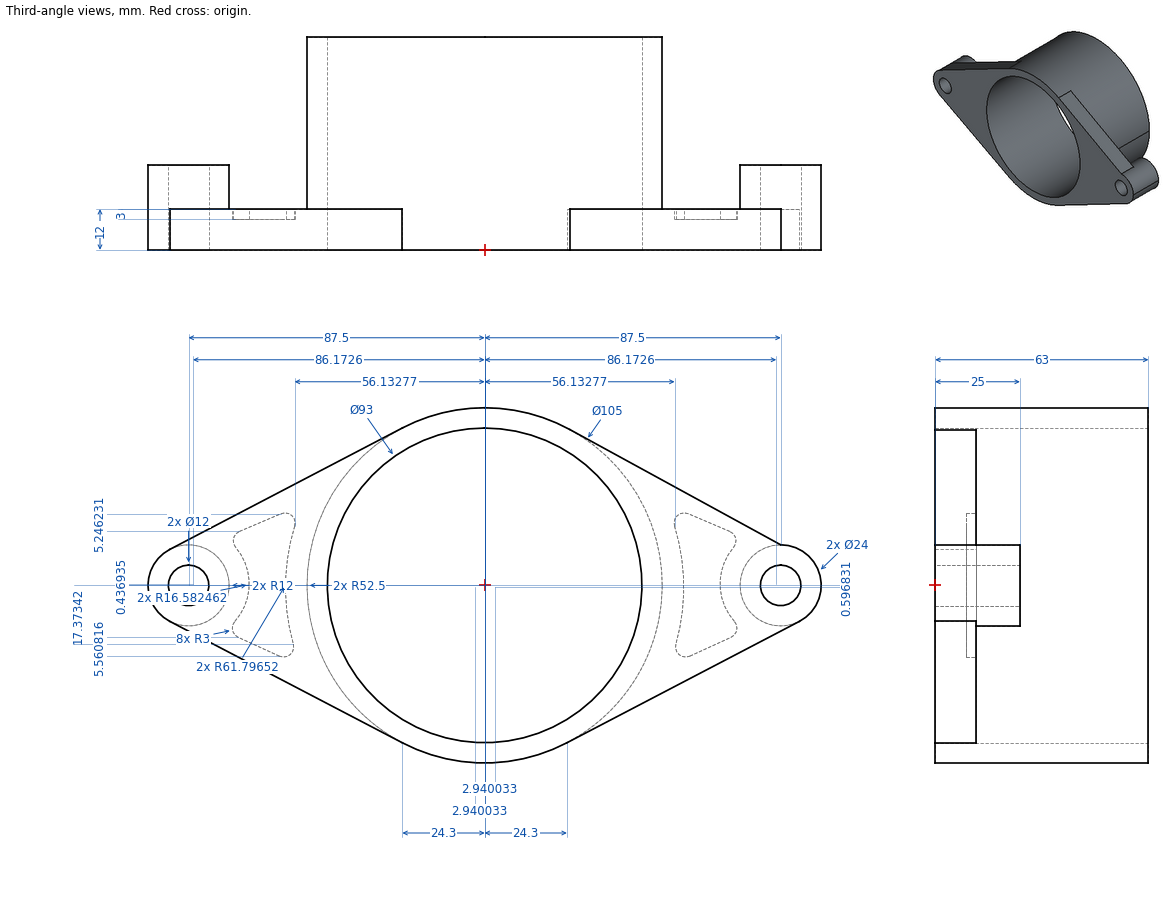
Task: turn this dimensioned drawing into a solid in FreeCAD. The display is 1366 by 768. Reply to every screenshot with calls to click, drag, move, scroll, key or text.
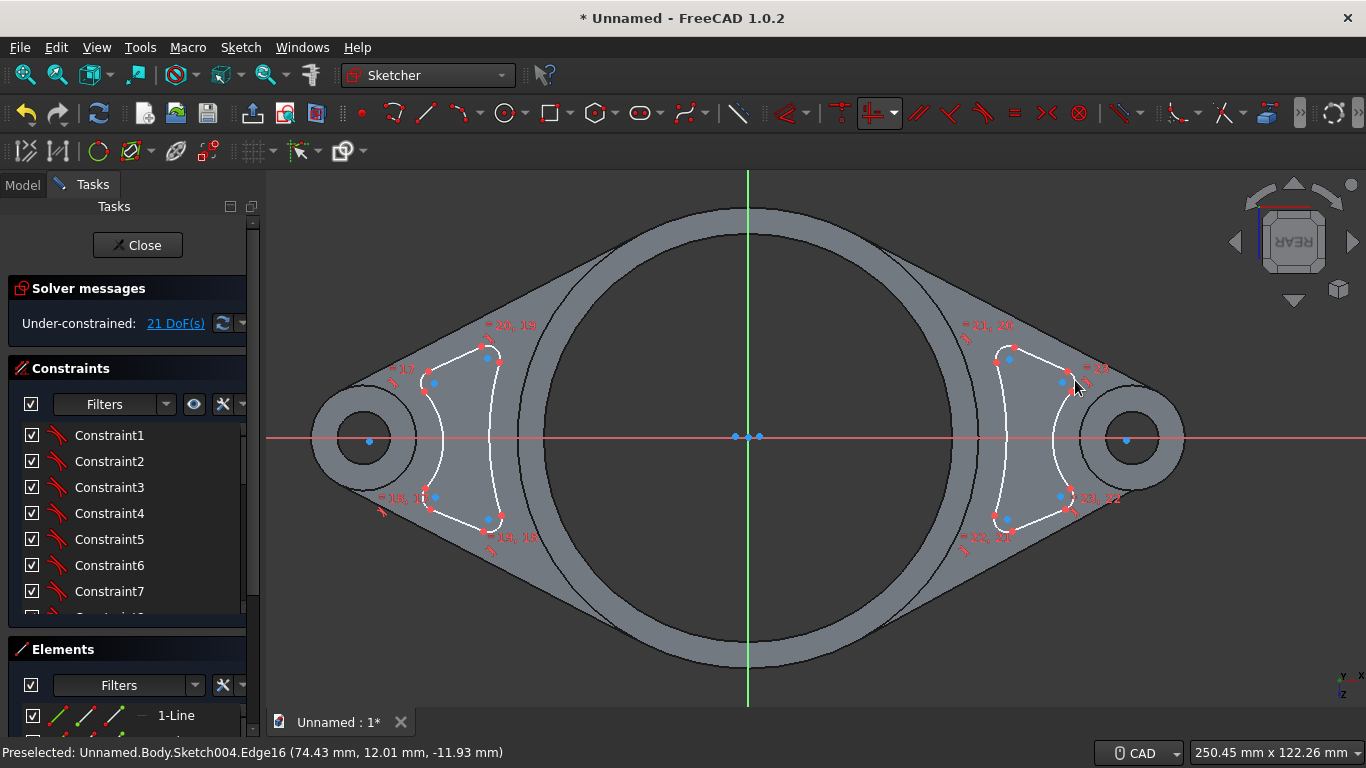
click(491, 408)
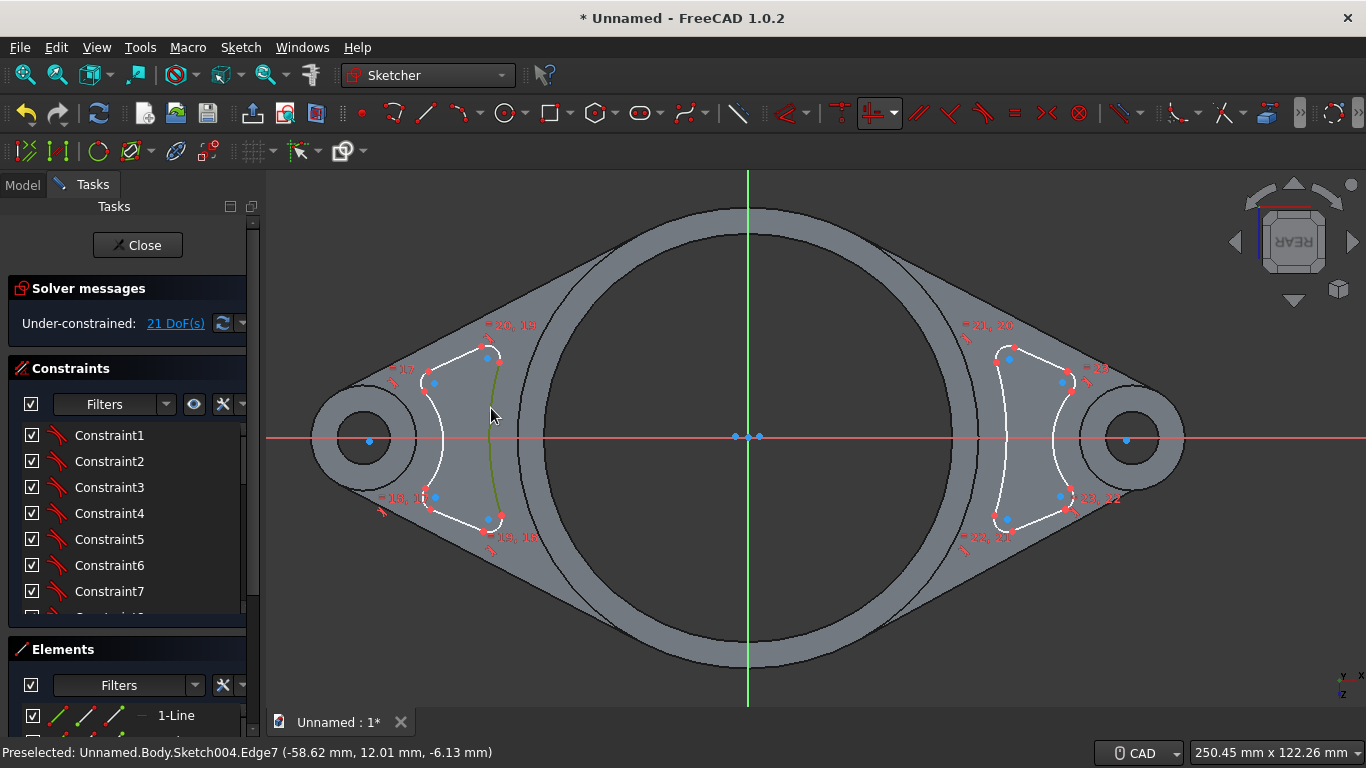
click(1004, 470)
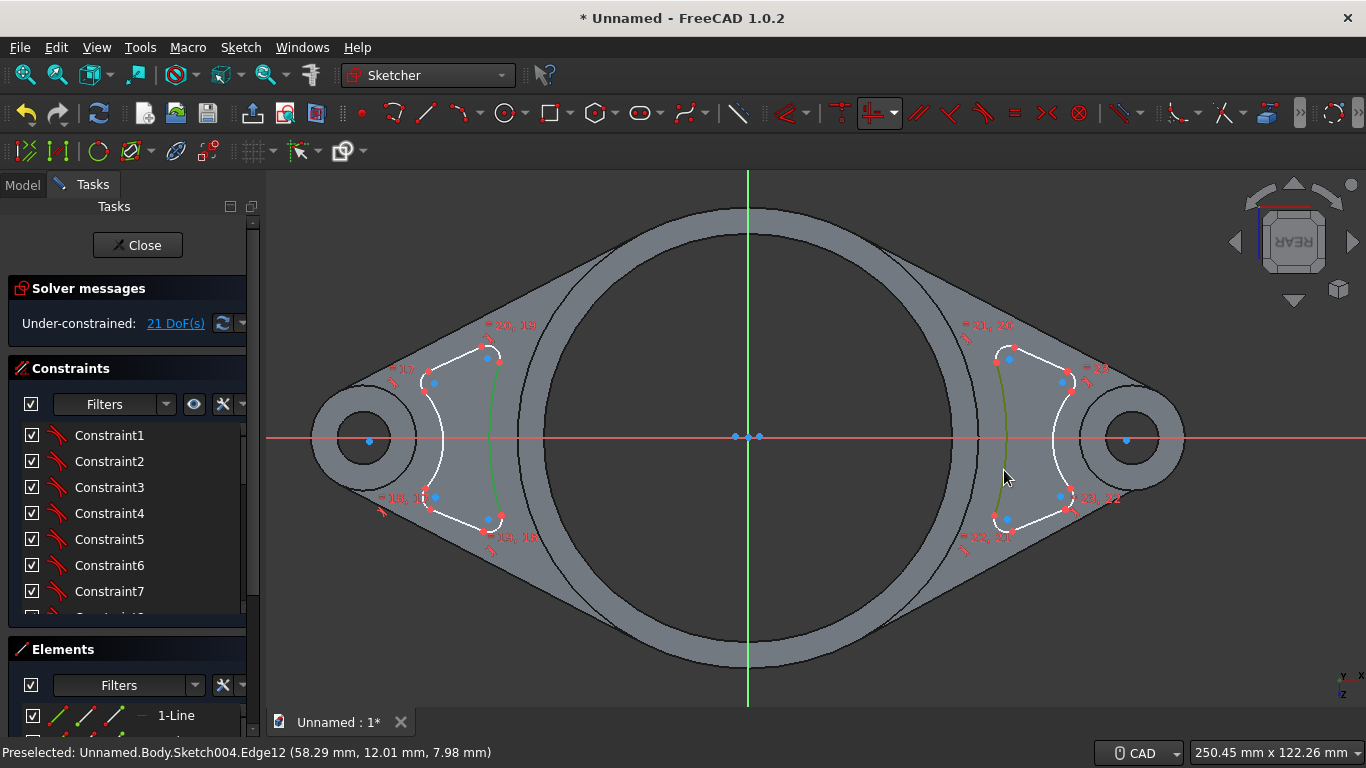
key(e)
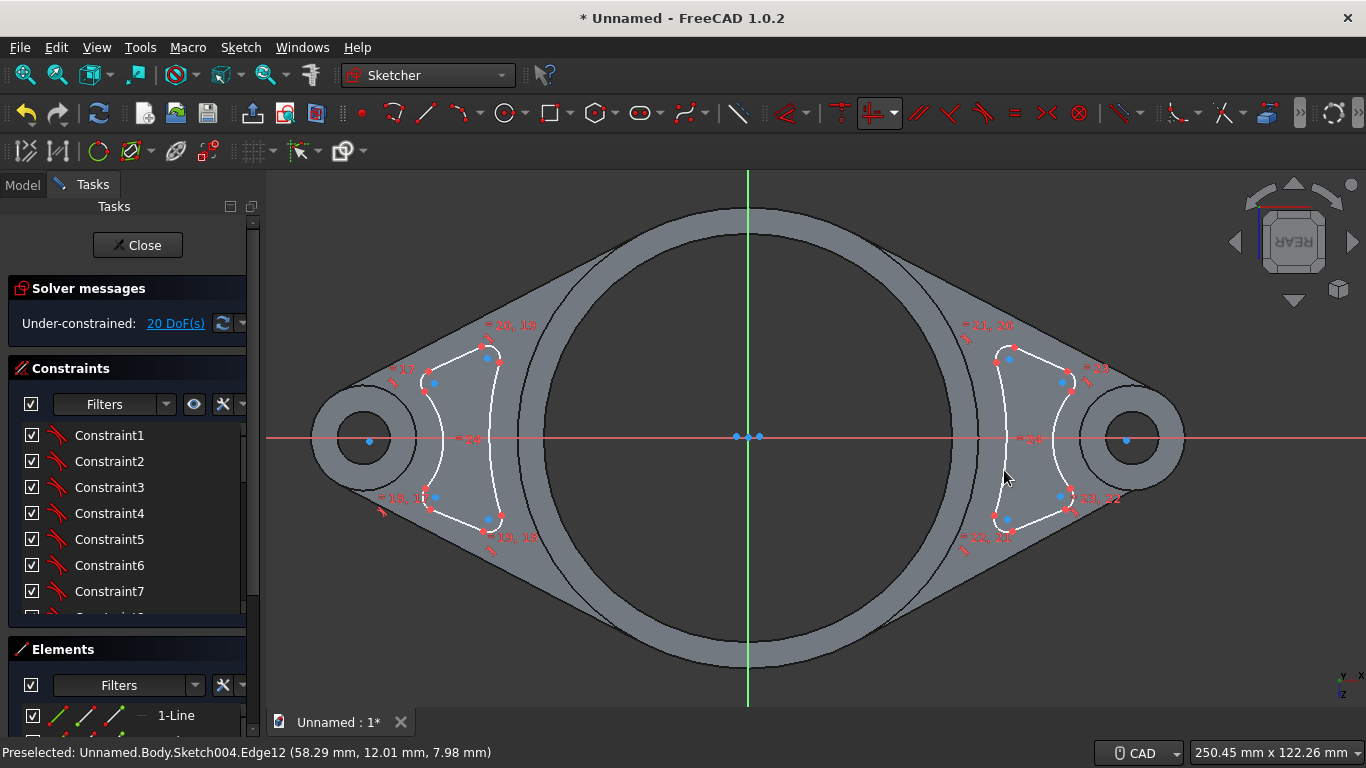
click(440, 461)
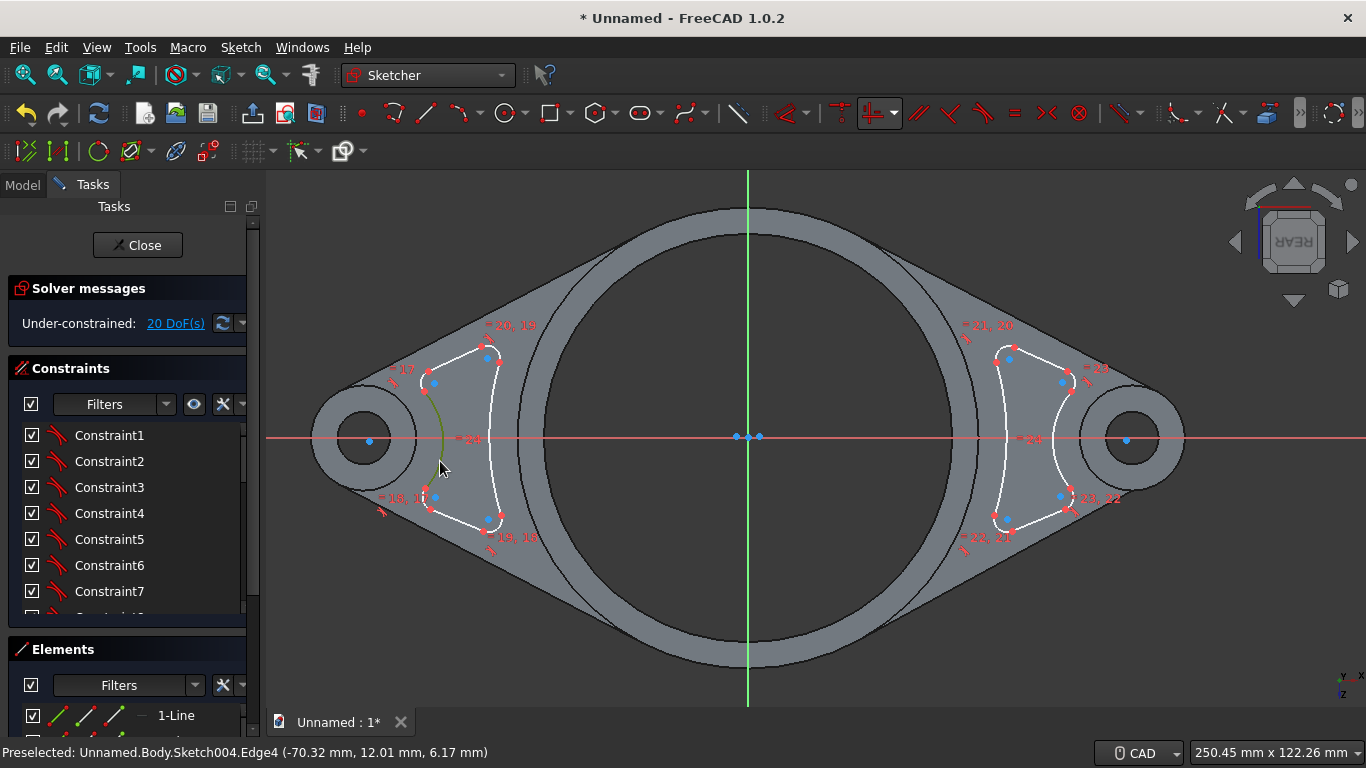
click(1056, 419)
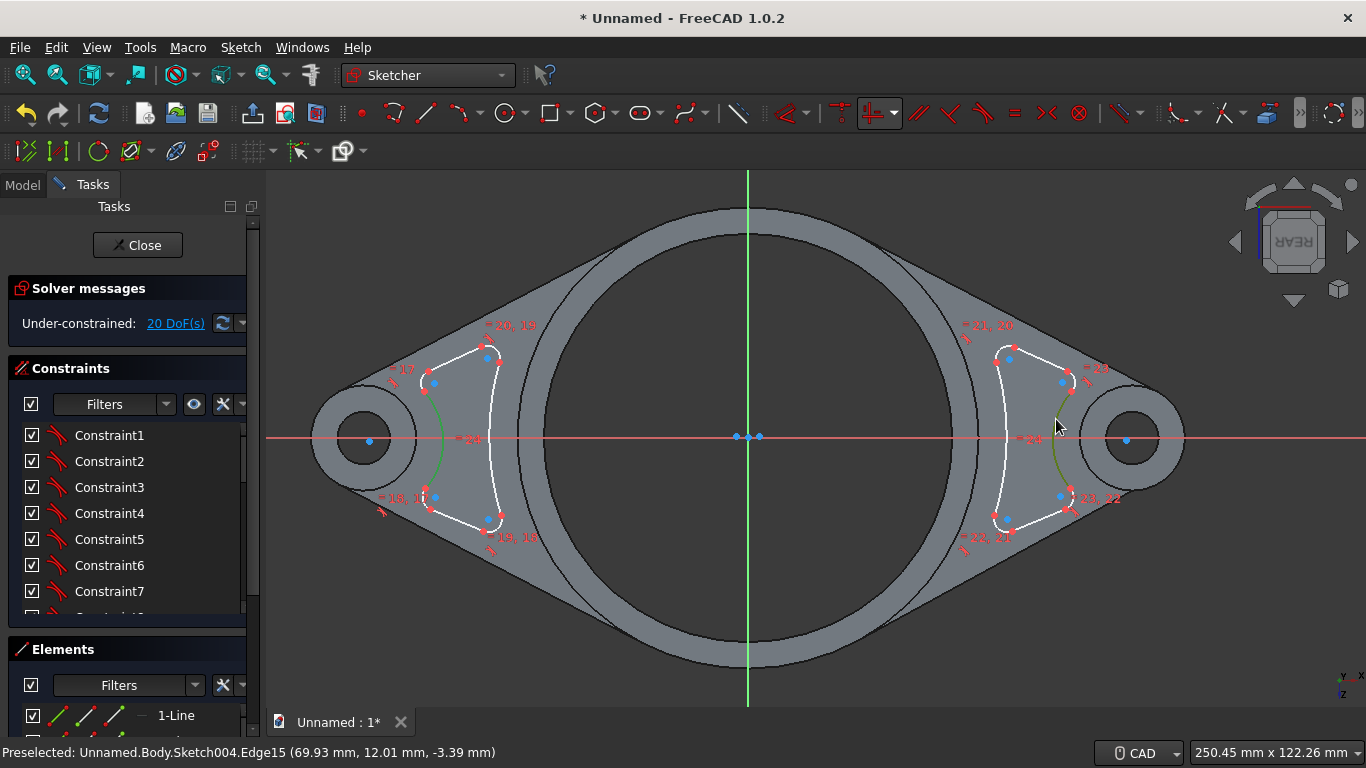
key(e)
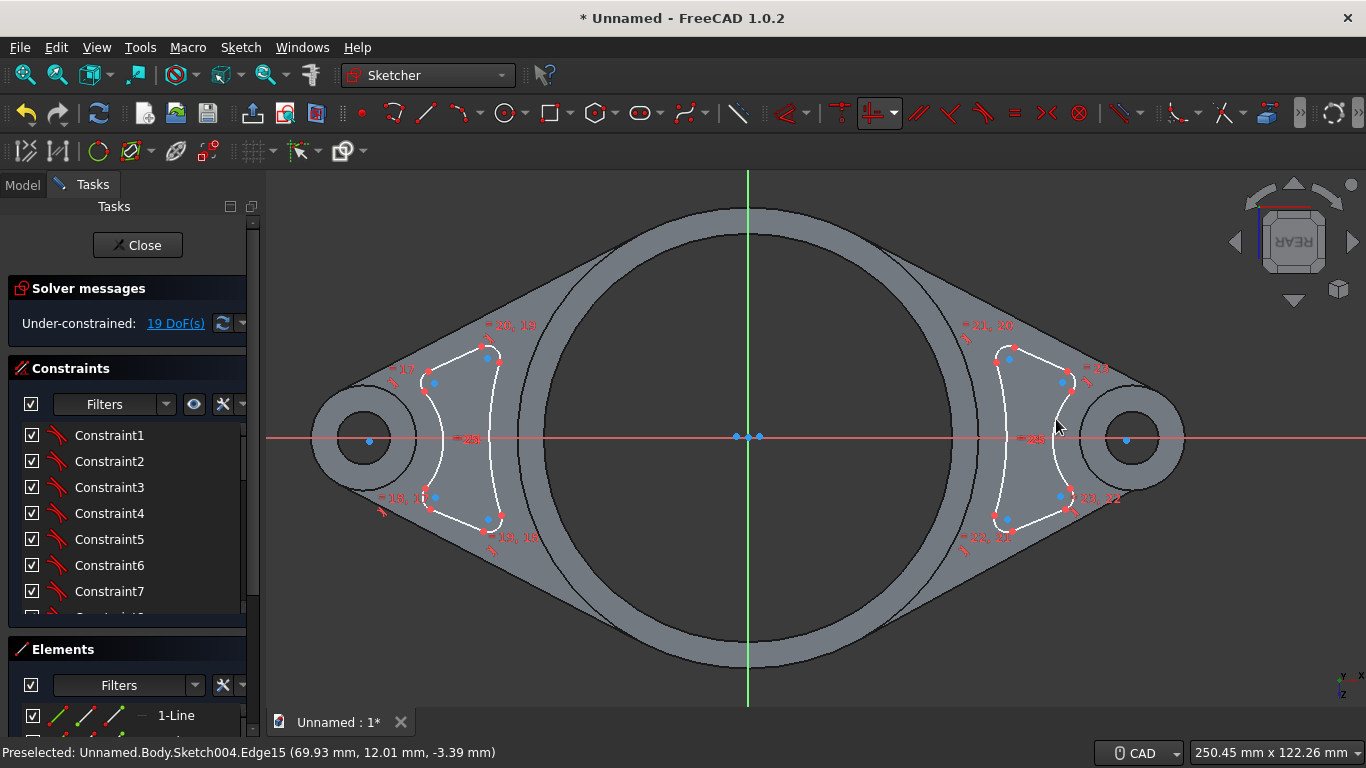
click(786, 114)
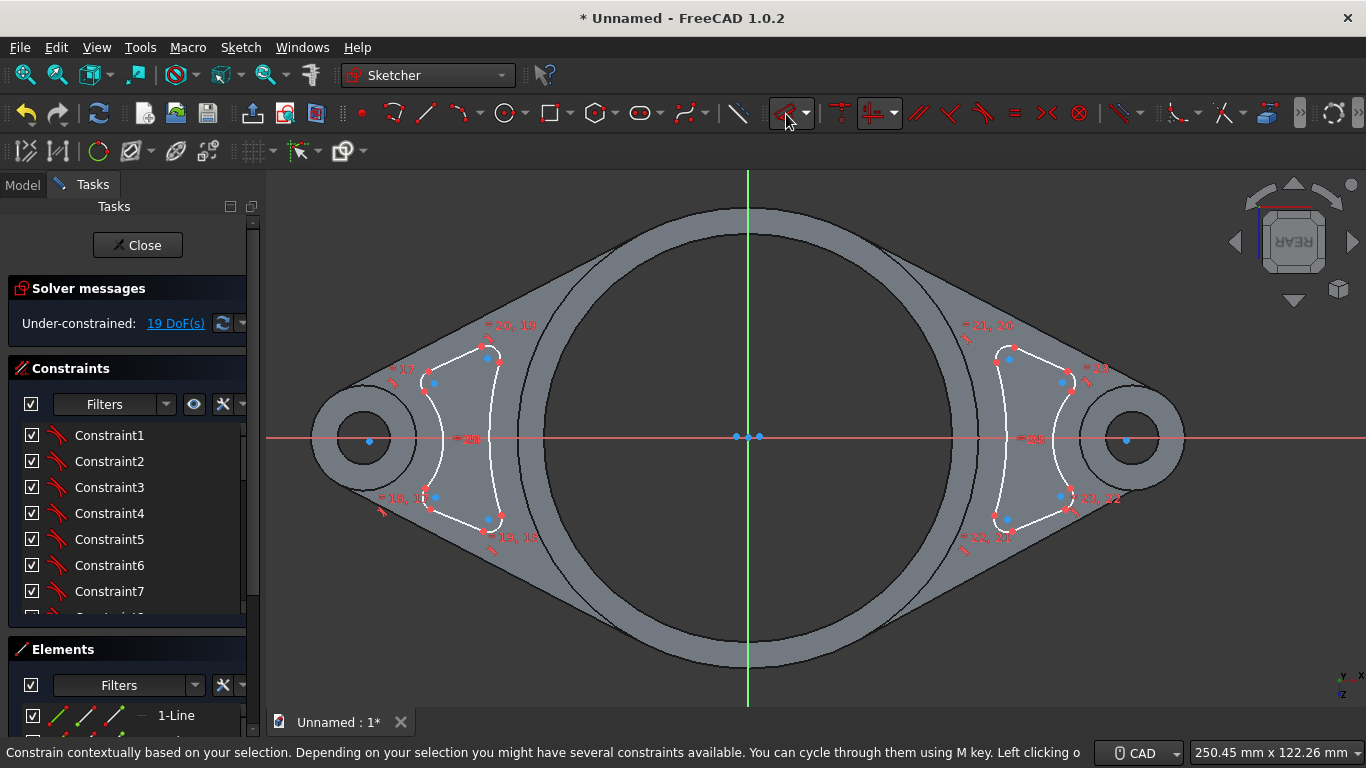
scroll(421, 381, up, 6)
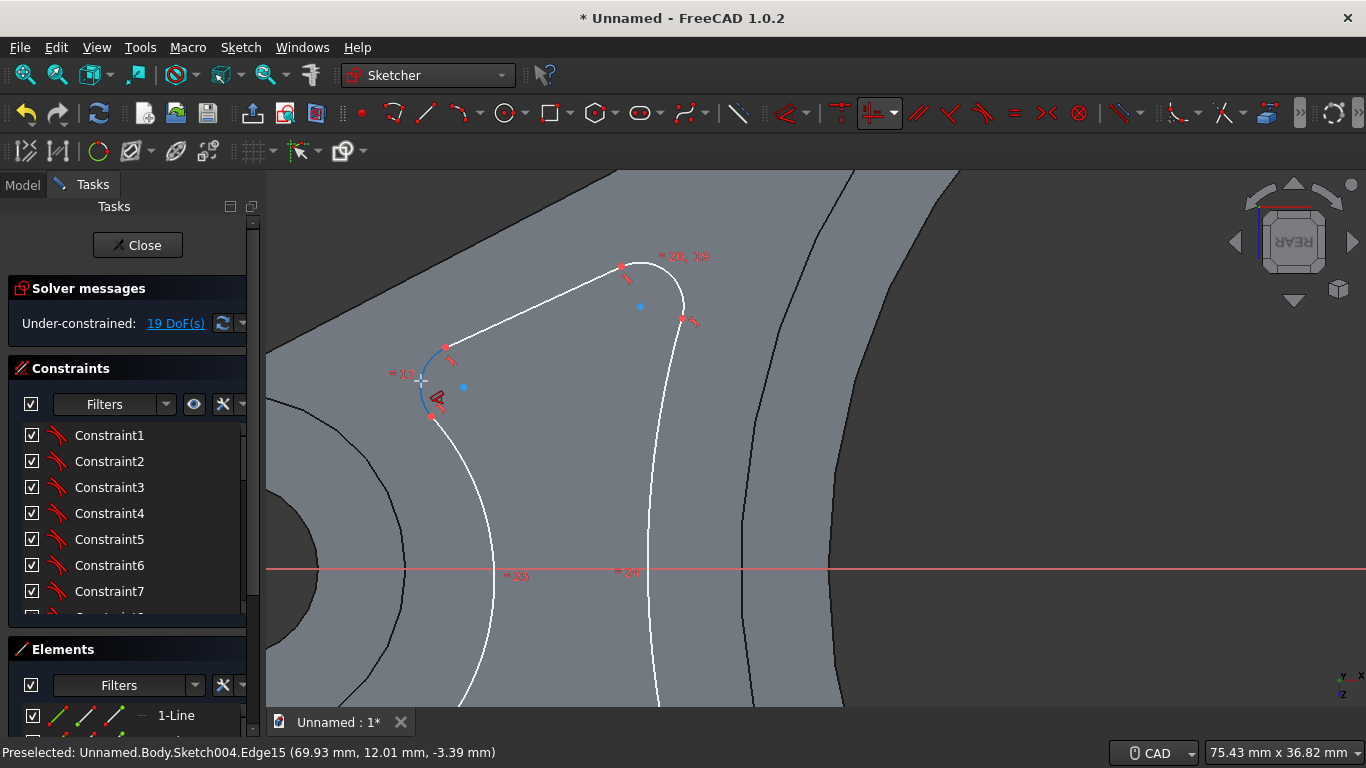
click(421, 379)
click(390, 373)